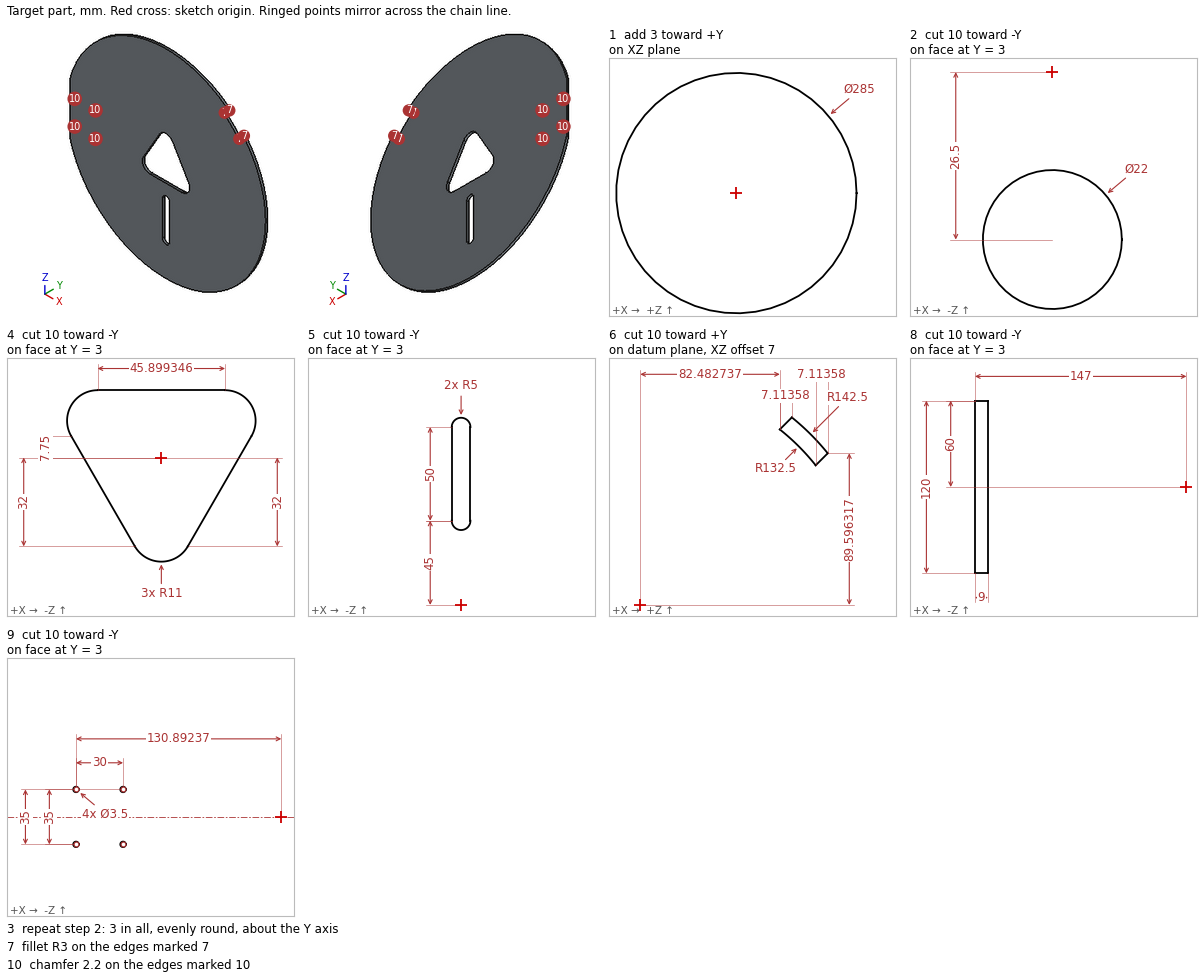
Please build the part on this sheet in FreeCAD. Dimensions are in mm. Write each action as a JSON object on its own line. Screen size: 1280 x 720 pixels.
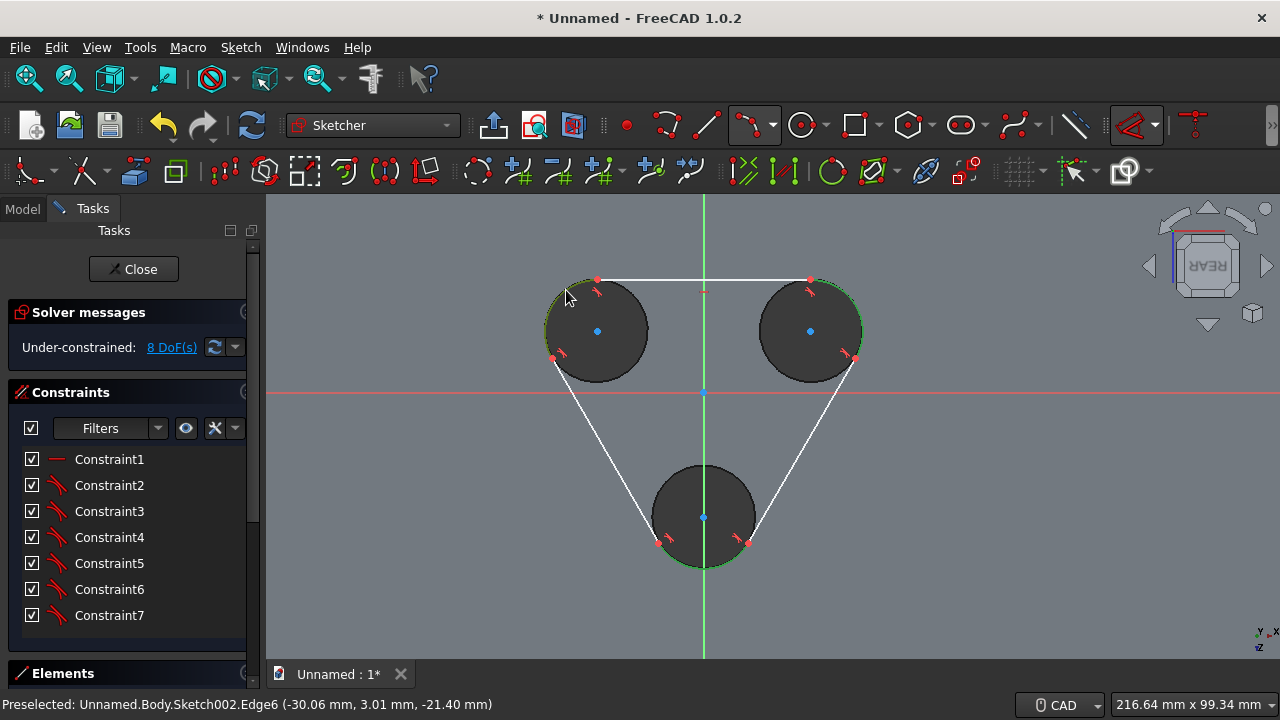
{"action": "key", "text": "e"}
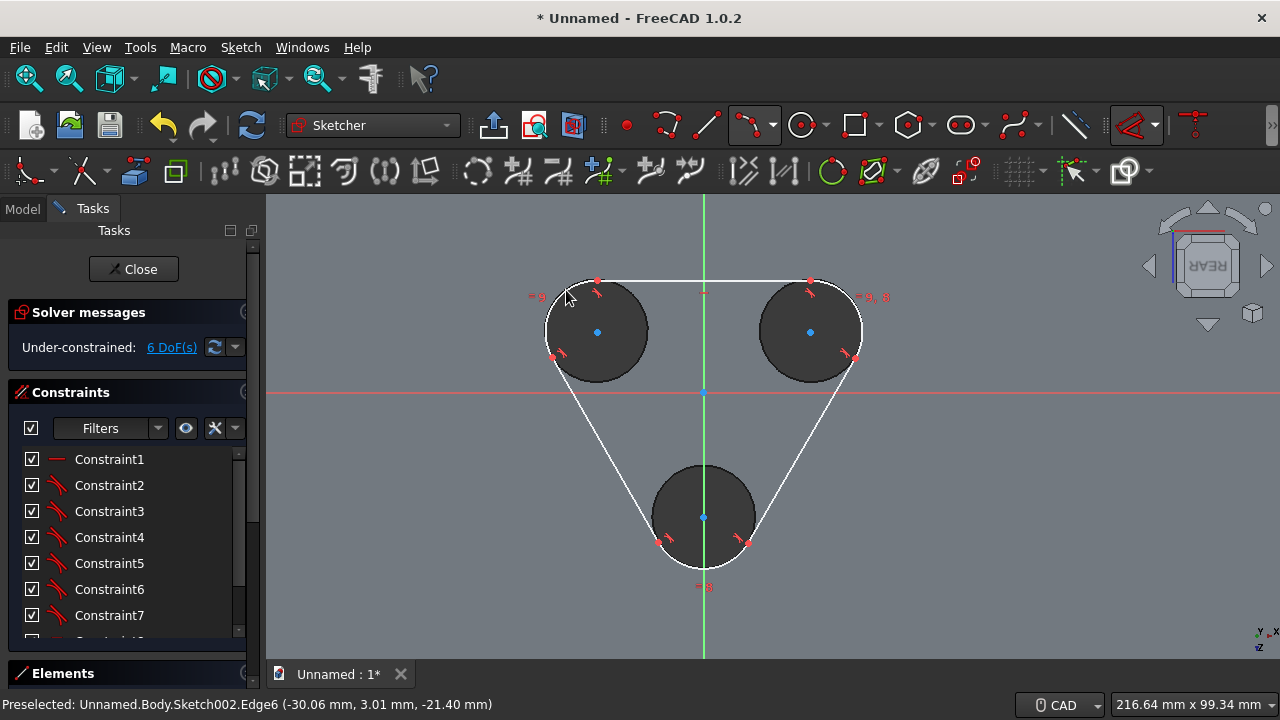
{"action": "left_click", "coordinate": [704, 517]}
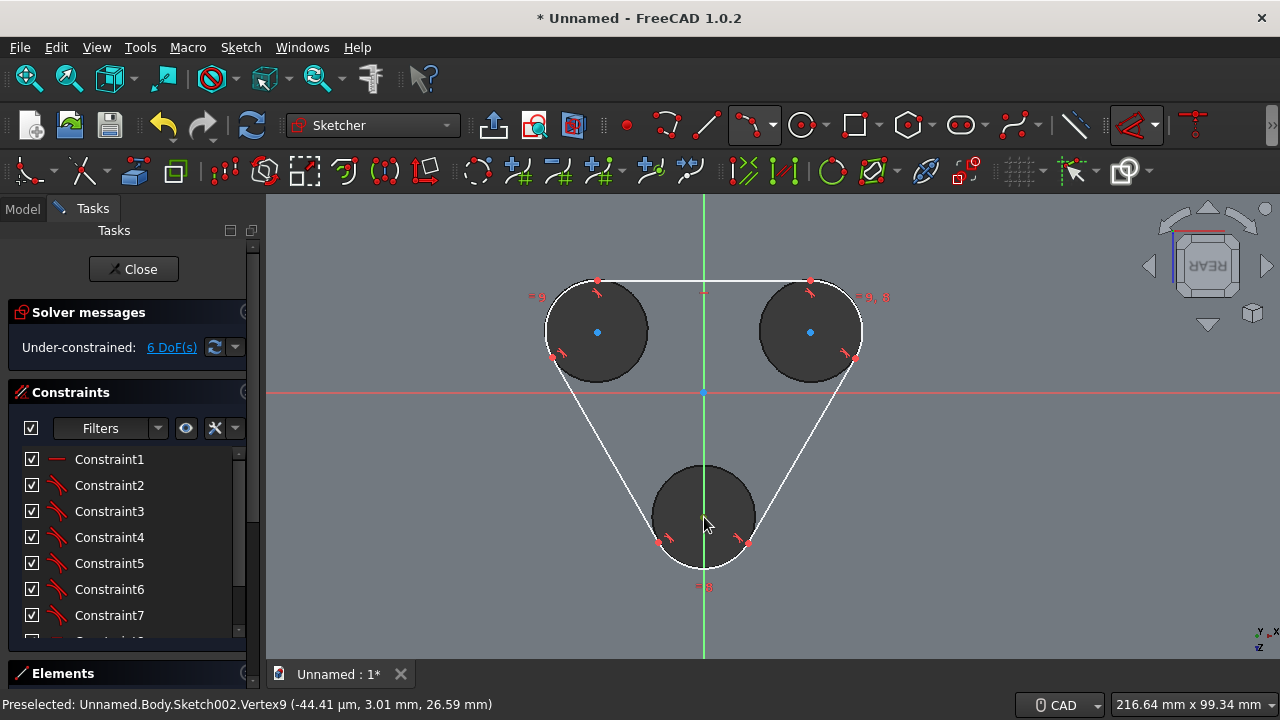
{"action": "left_click", "coordinate": [704, 602]}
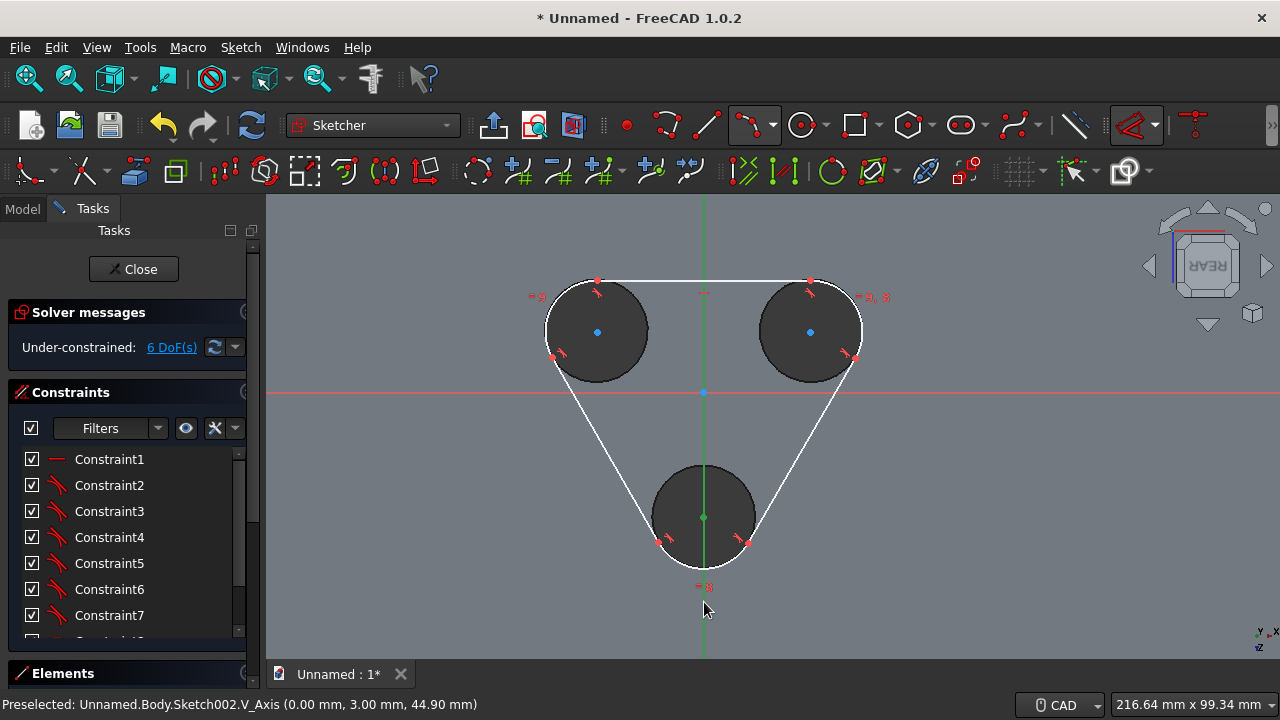
{"action": "left_click", "coordinate": [1194, 126]}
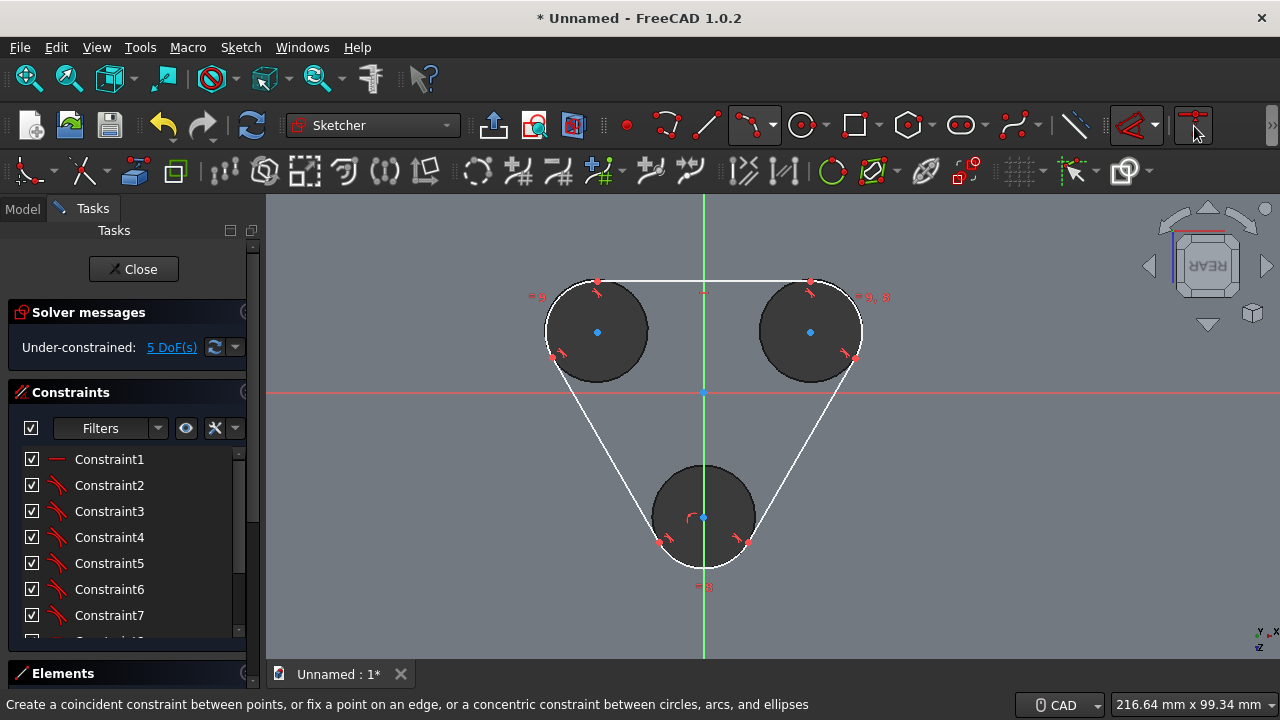
{"action": "left_click", "coordinate": [683, 564]}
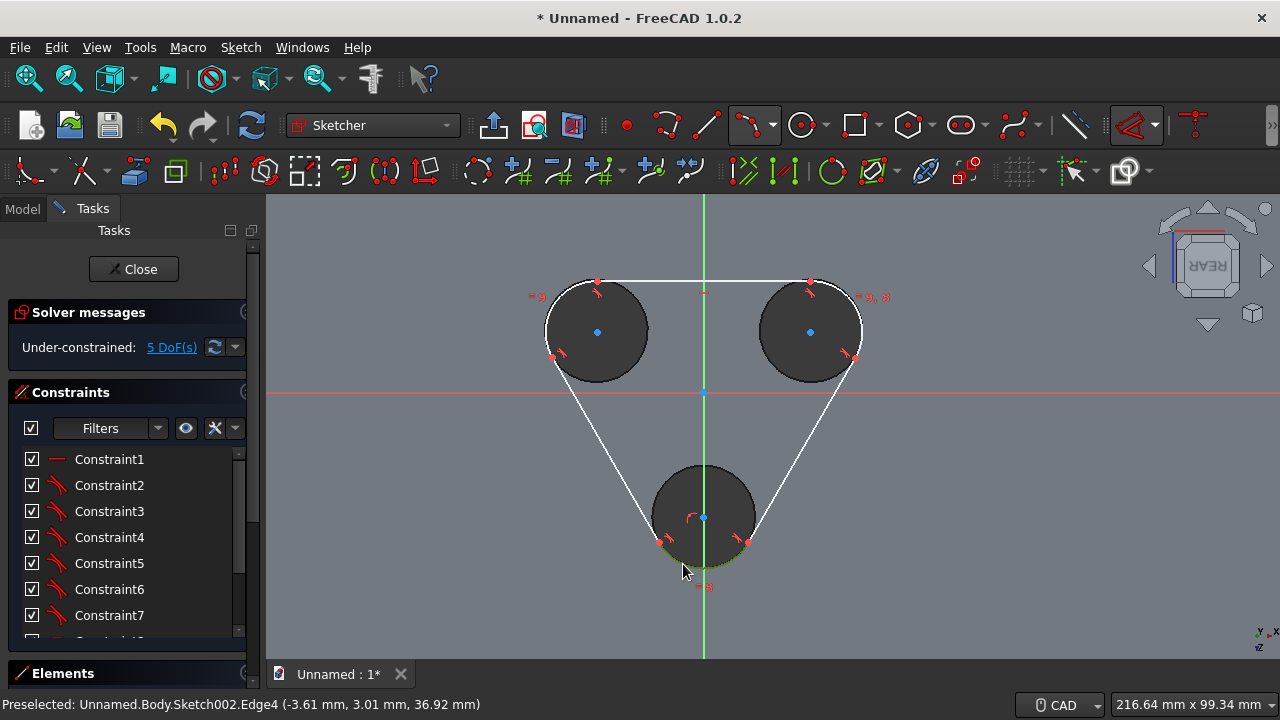
{"action": "key", "text": "k r"}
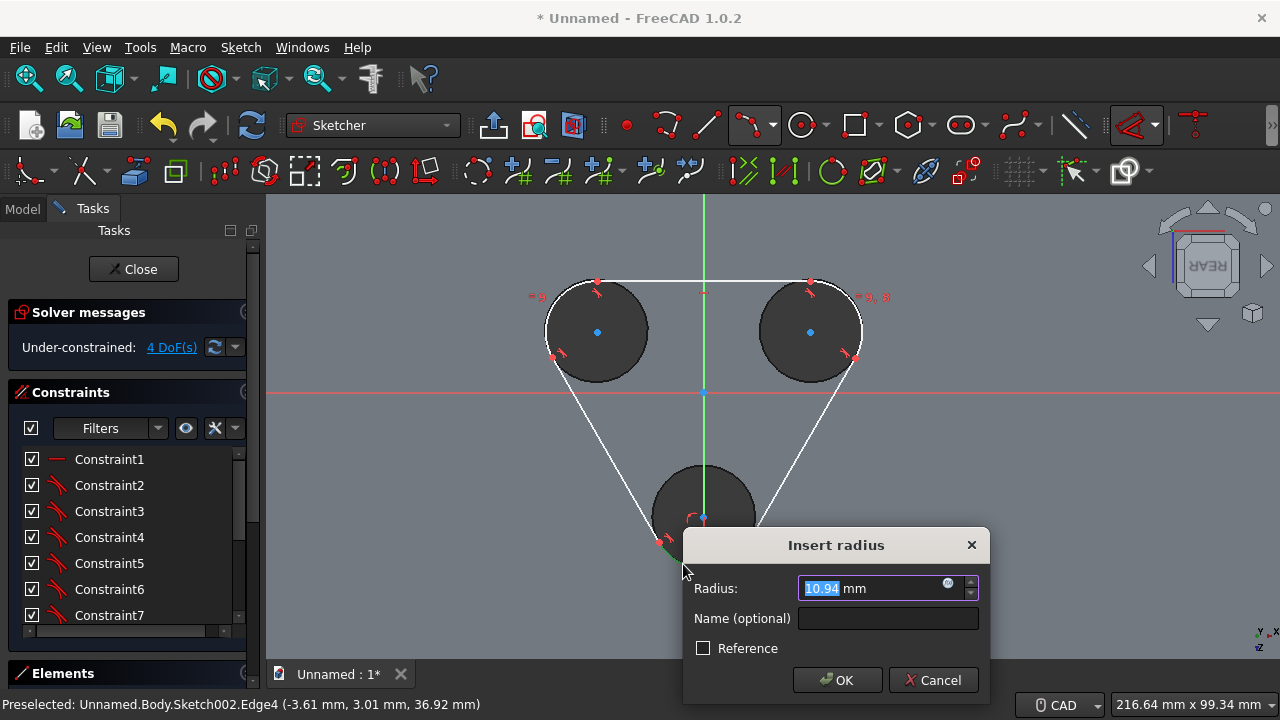
{"action": "type", "text": "11"}
{"action": "key", "text": "Return"}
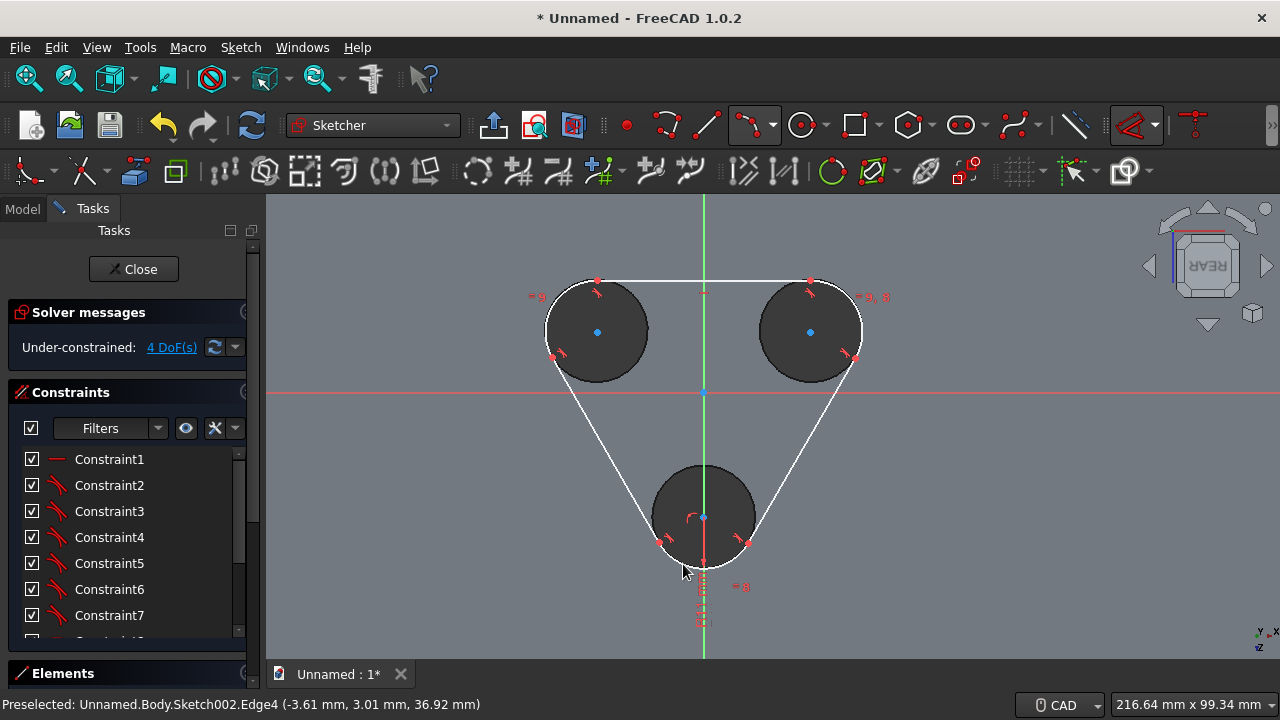
{"action": "left_click", "coordinate": [659, 543]}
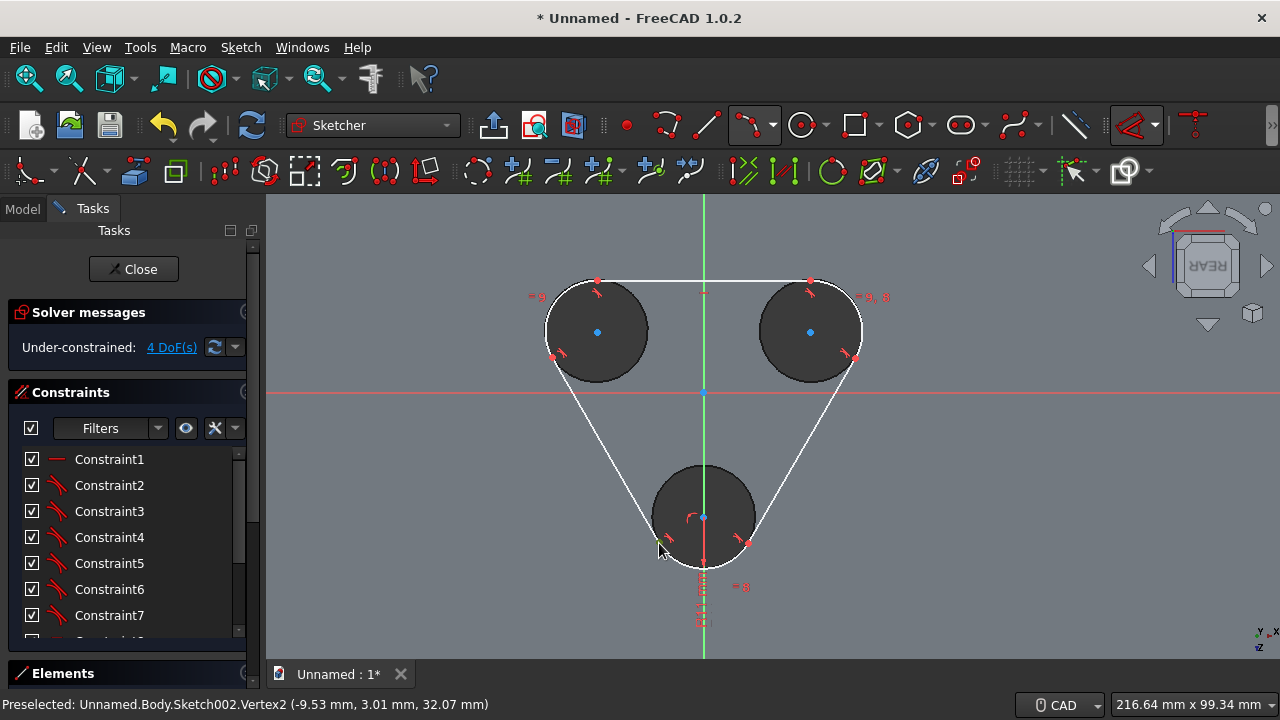
{"action": "left_click", "coordinate": [1158, 126]}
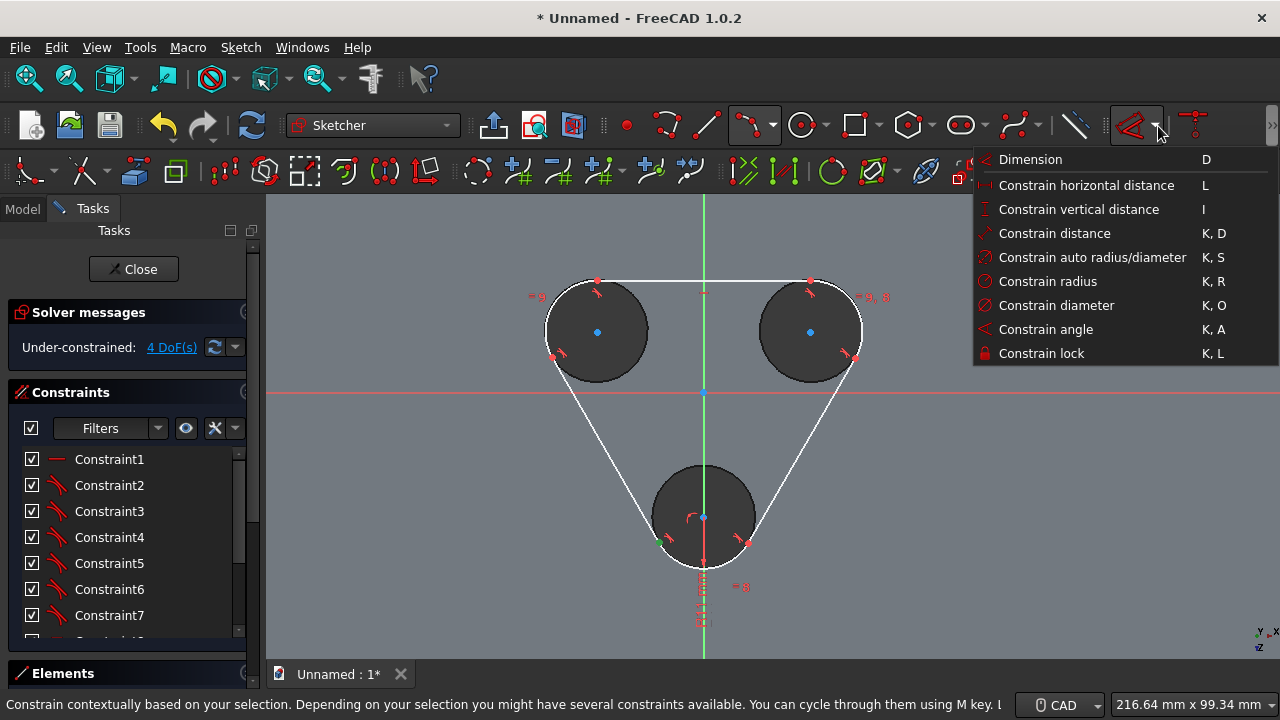
{"action": "left_click", "coordinate": [1126, 209]}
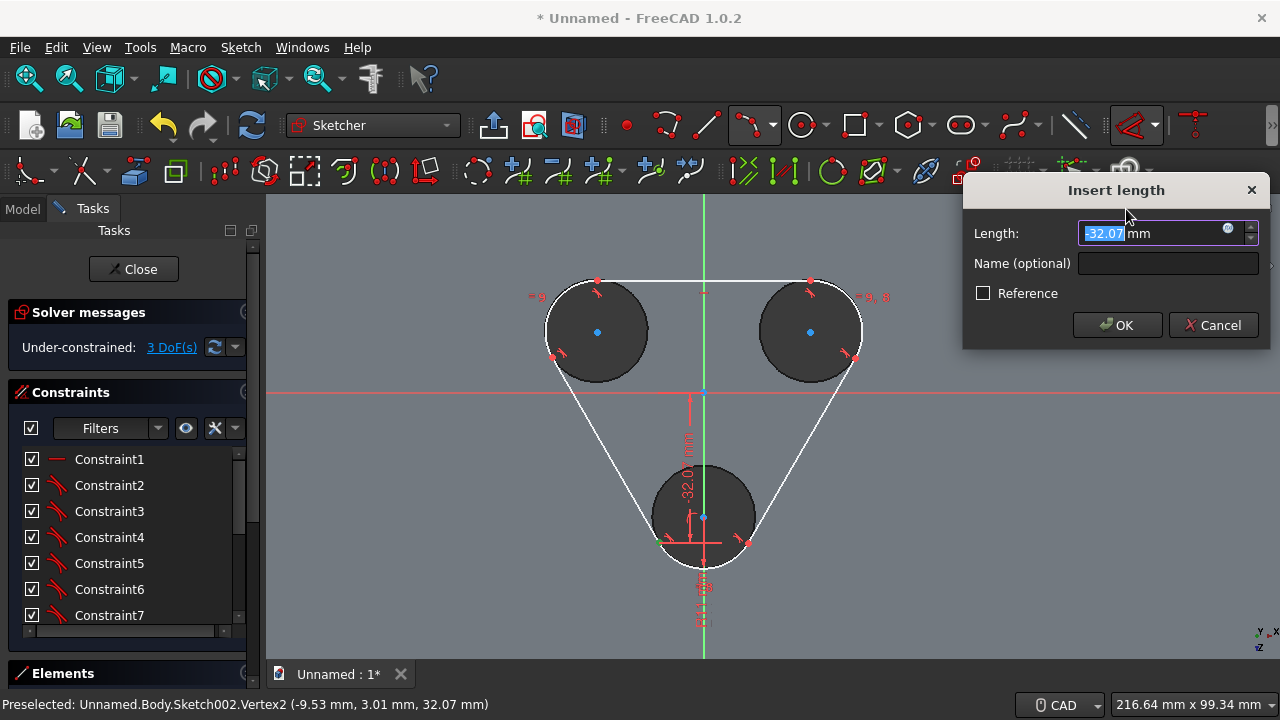
{"action": "type", "text": "-32"}
{"action": "key", "text": "Return"}